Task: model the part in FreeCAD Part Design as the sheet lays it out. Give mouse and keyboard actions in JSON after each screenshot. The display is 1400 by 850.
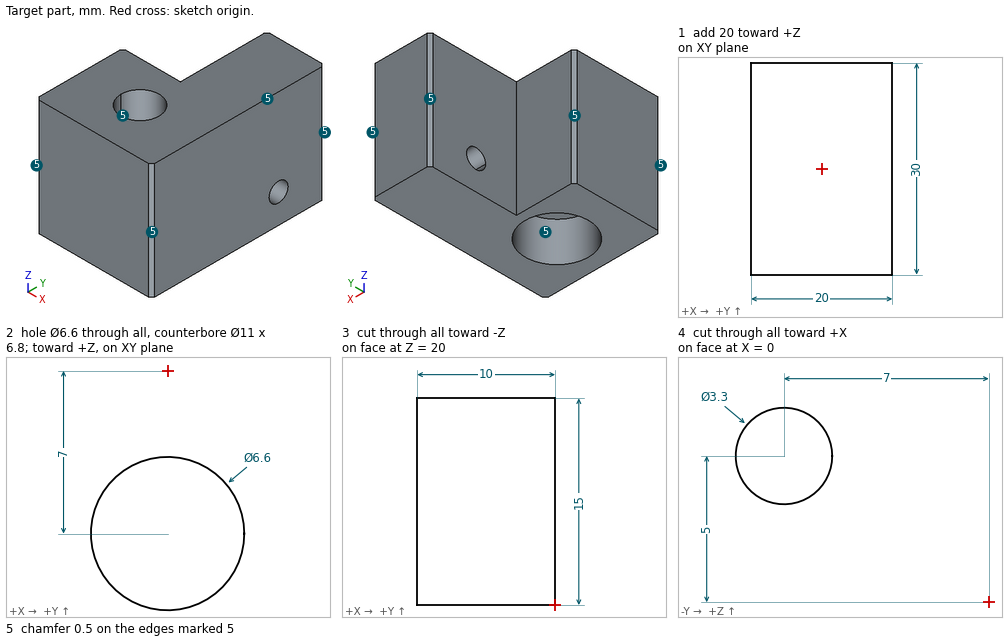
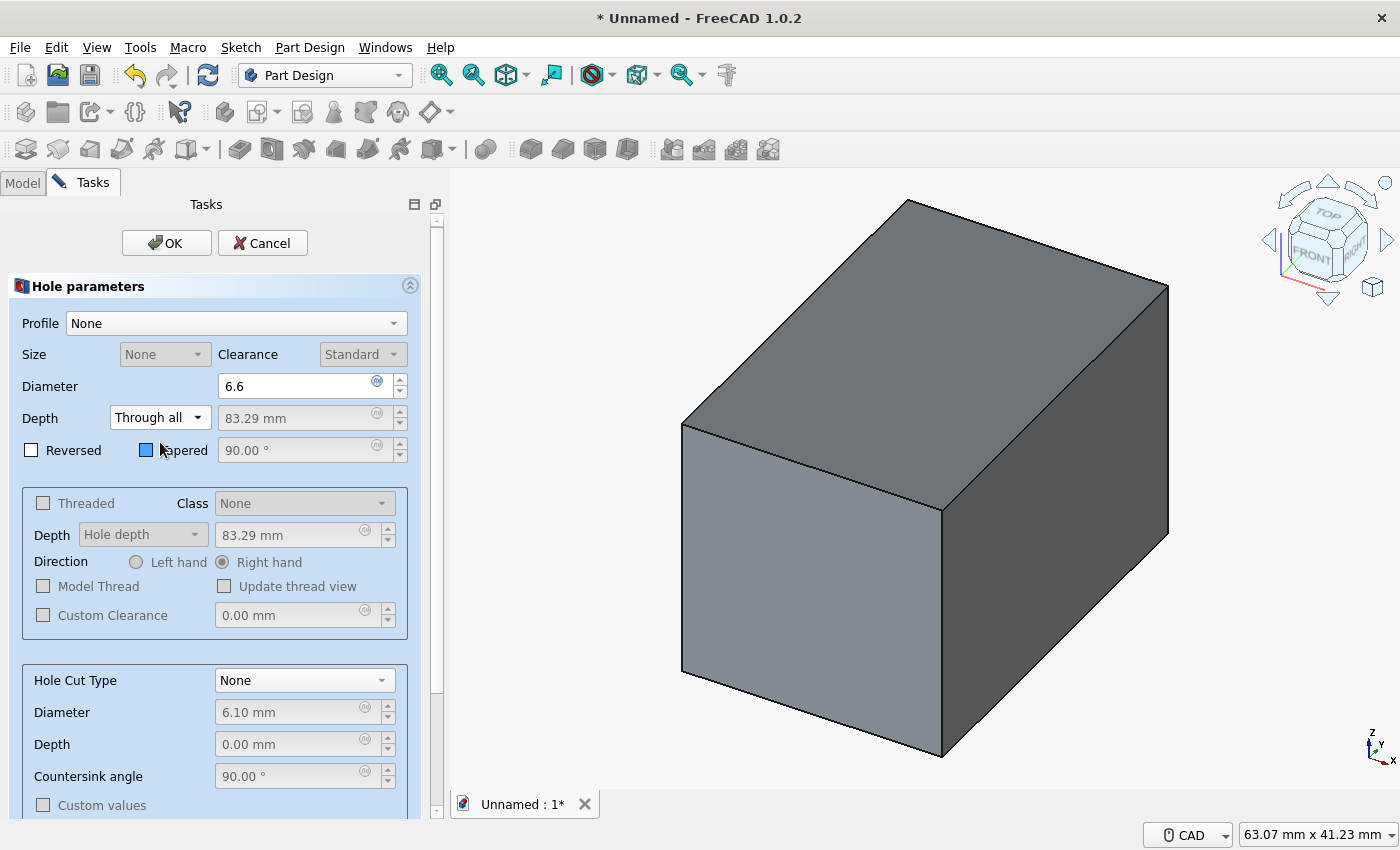
{"action": "left_click", "coordinate": [30, 450]}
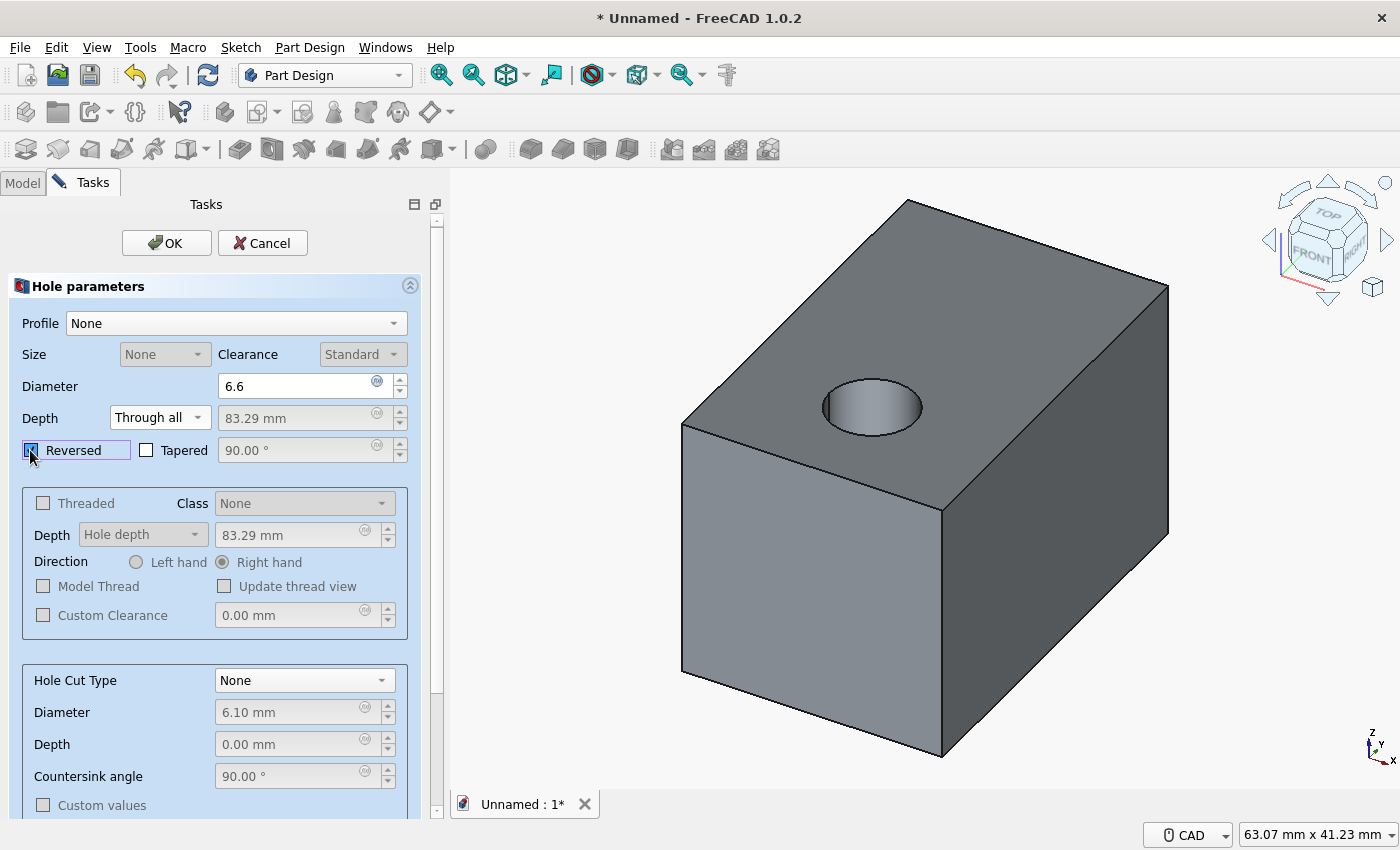
{"action": "left_click", "coordinate": [306, 680]}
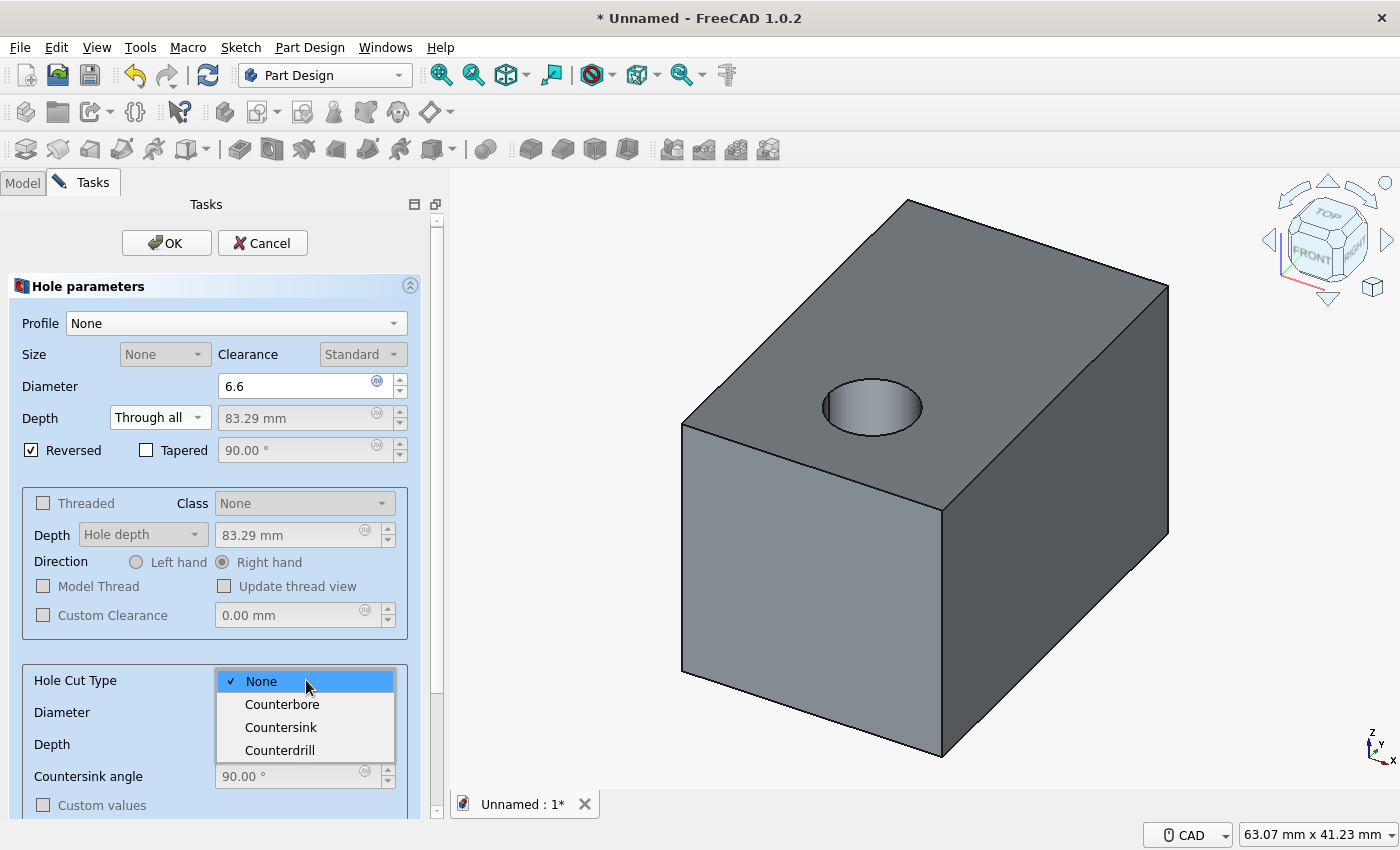
{"action": "left_click", "coordinate": [304, 704]}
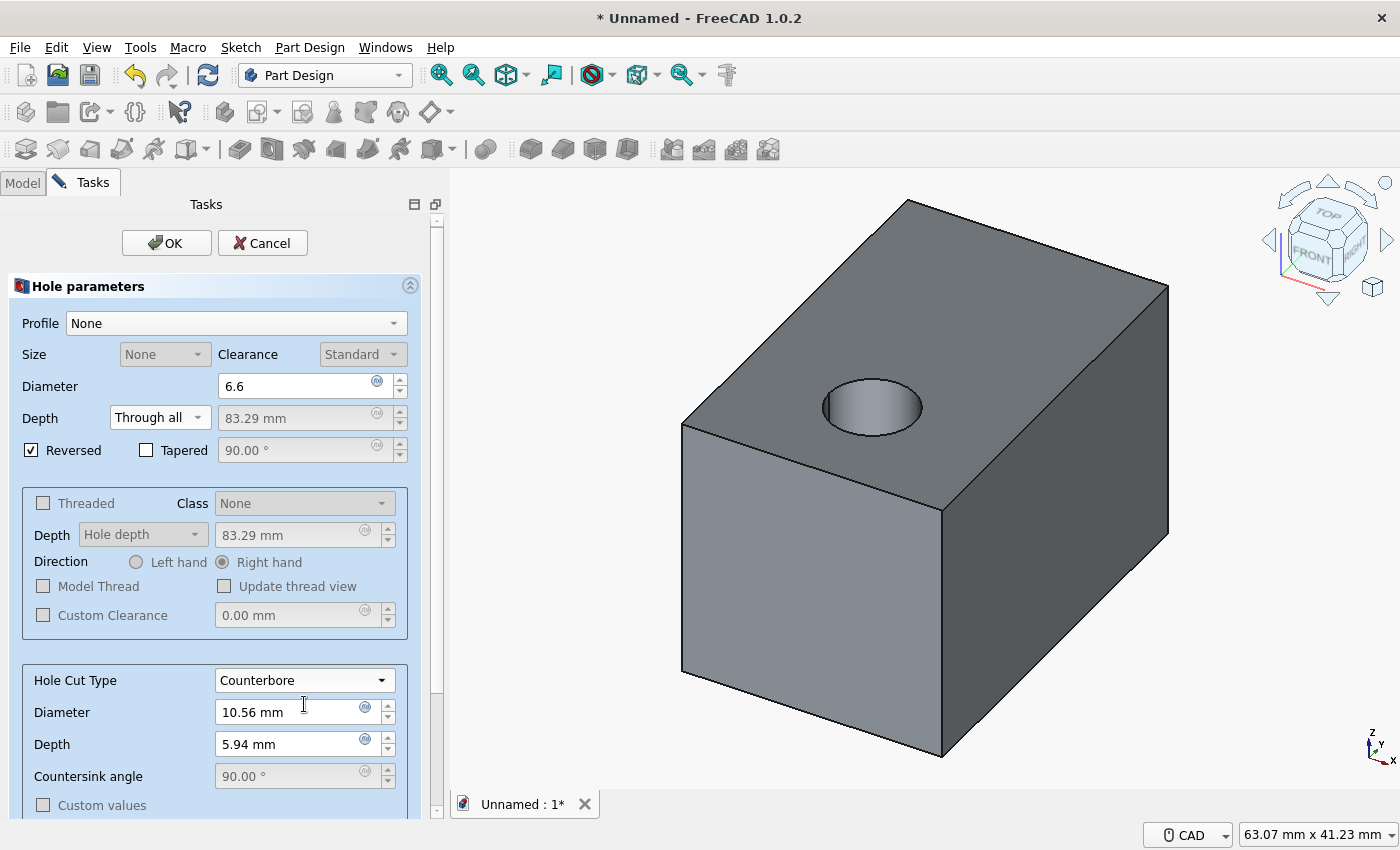
{"action": "triple_click", "coordinate": [298, 712]}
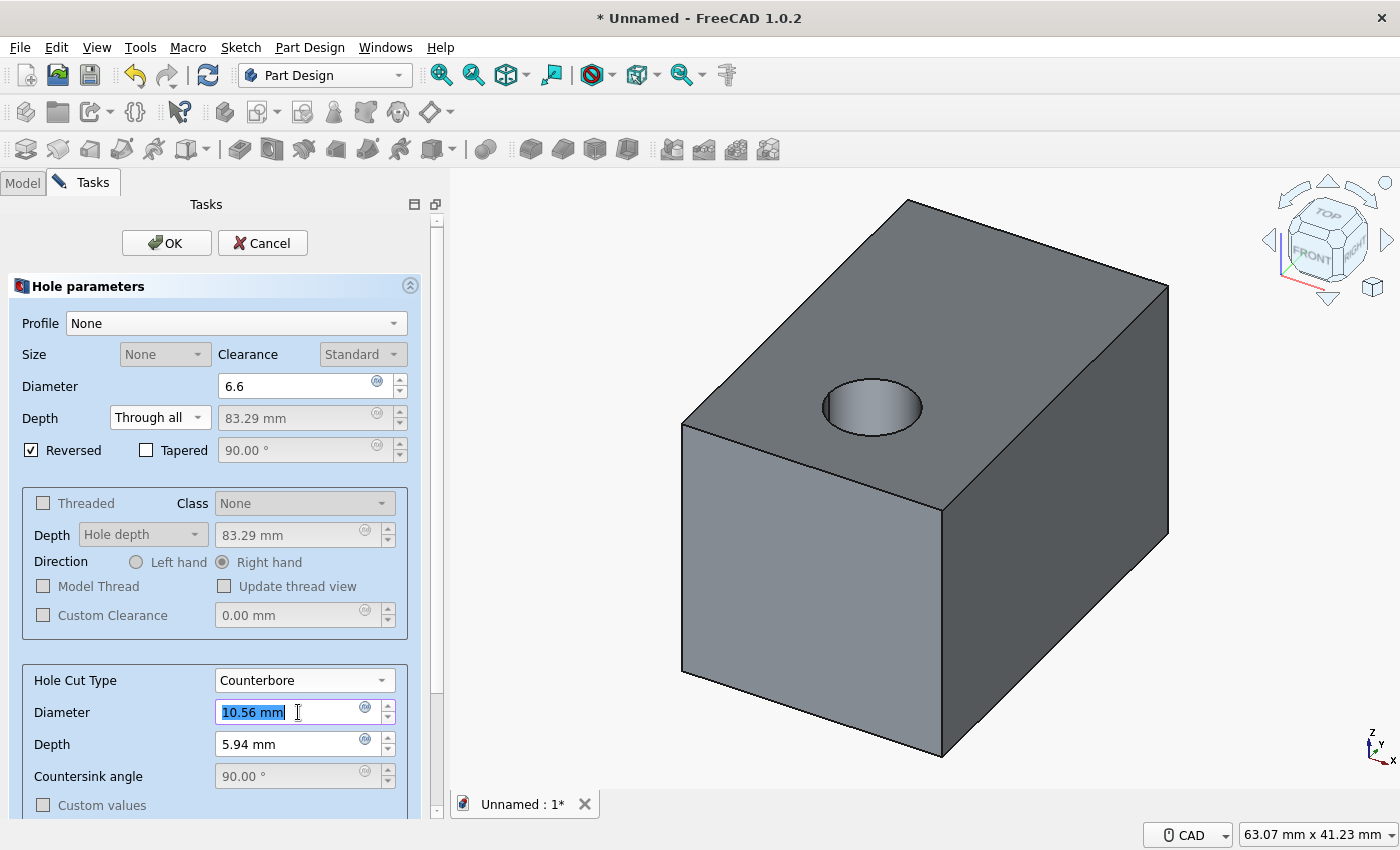
{"action": "type", "text": "11"}
{"action": "key", "text": "Tab"}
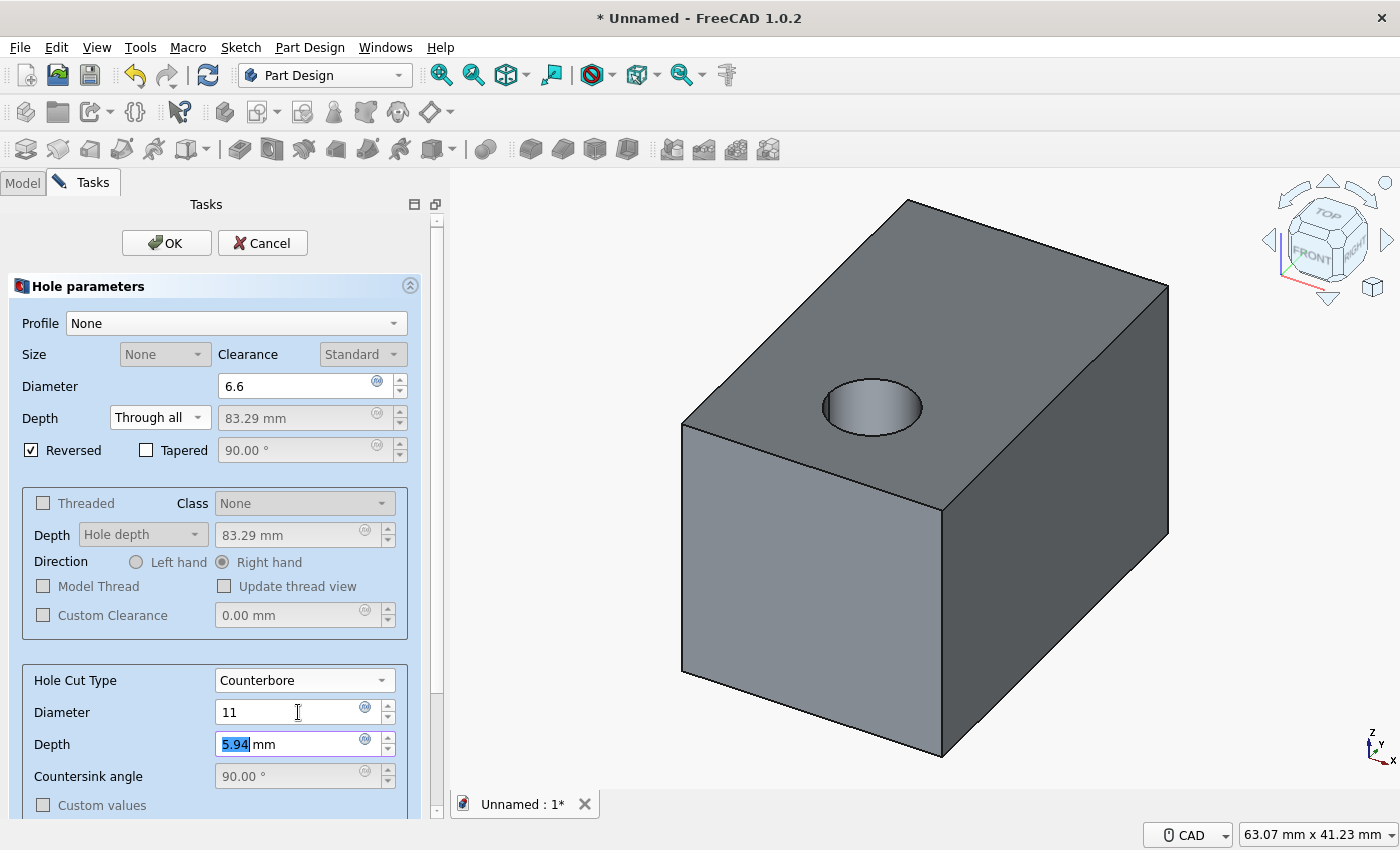
{"action": "type", "text": "6.8"}
{"action": "key", "text": "Tab"}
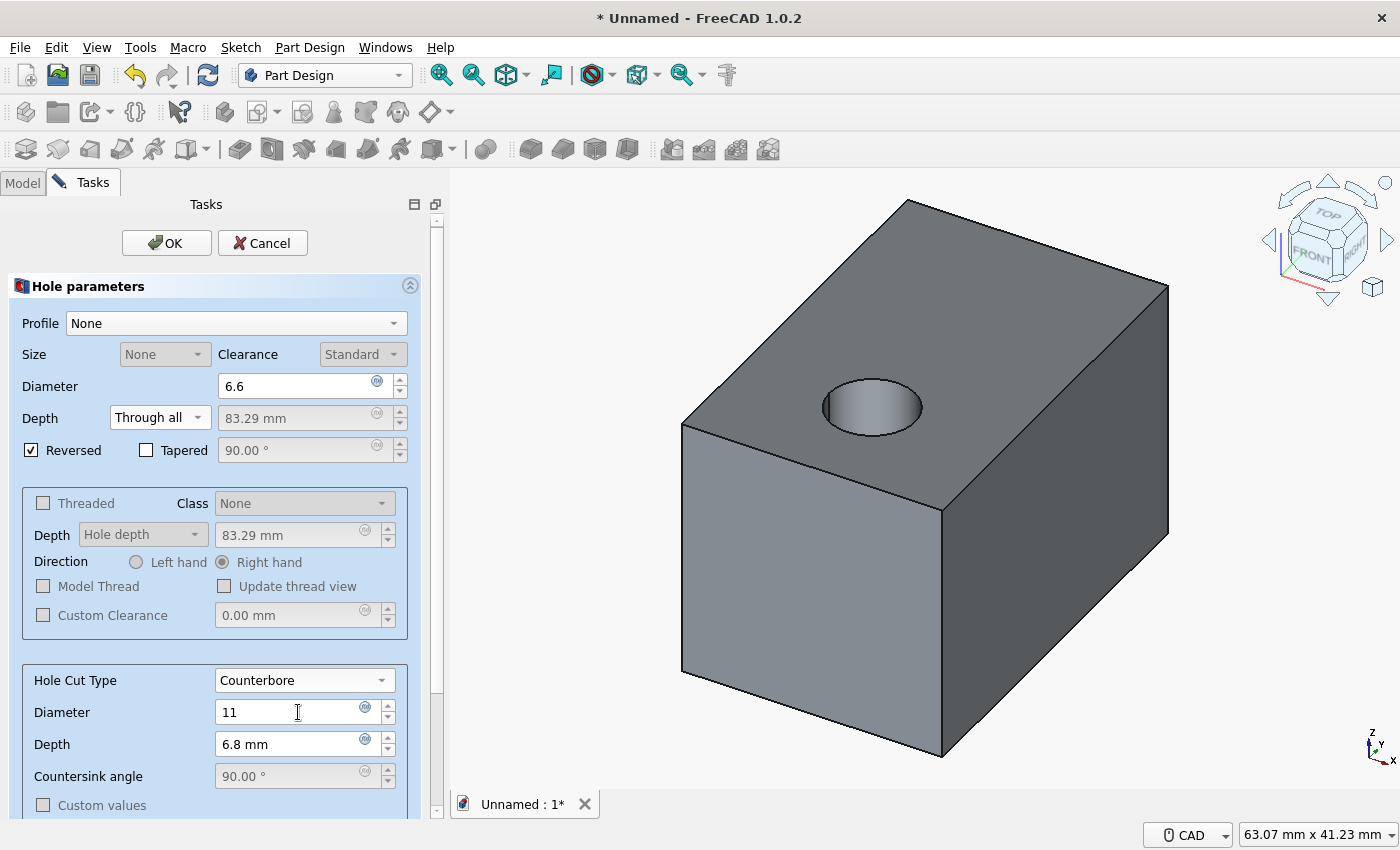
{"action": "left_click", "coordinate": [167, 243]}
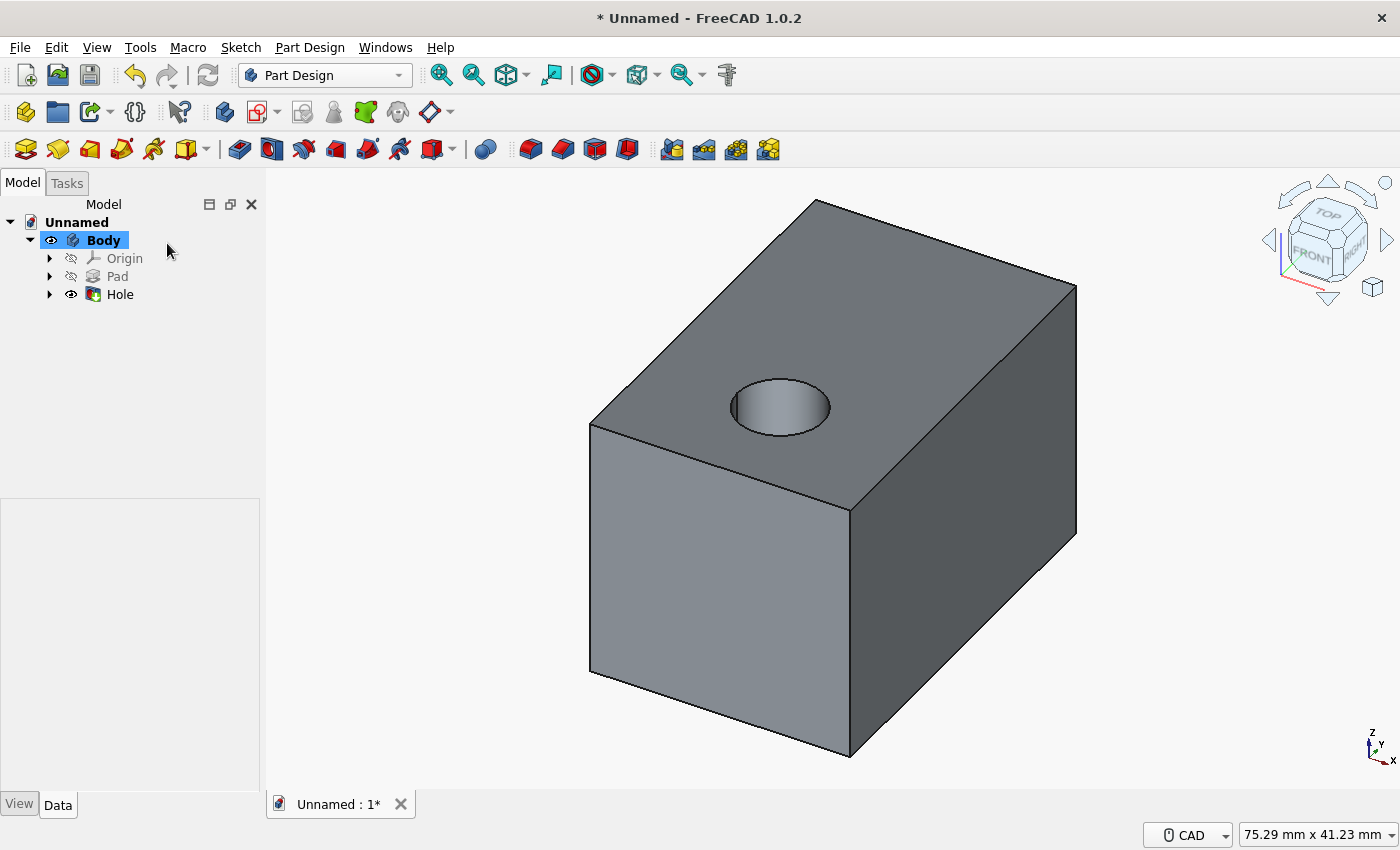
{"action": "left_click", "coordinate": [865, 322]}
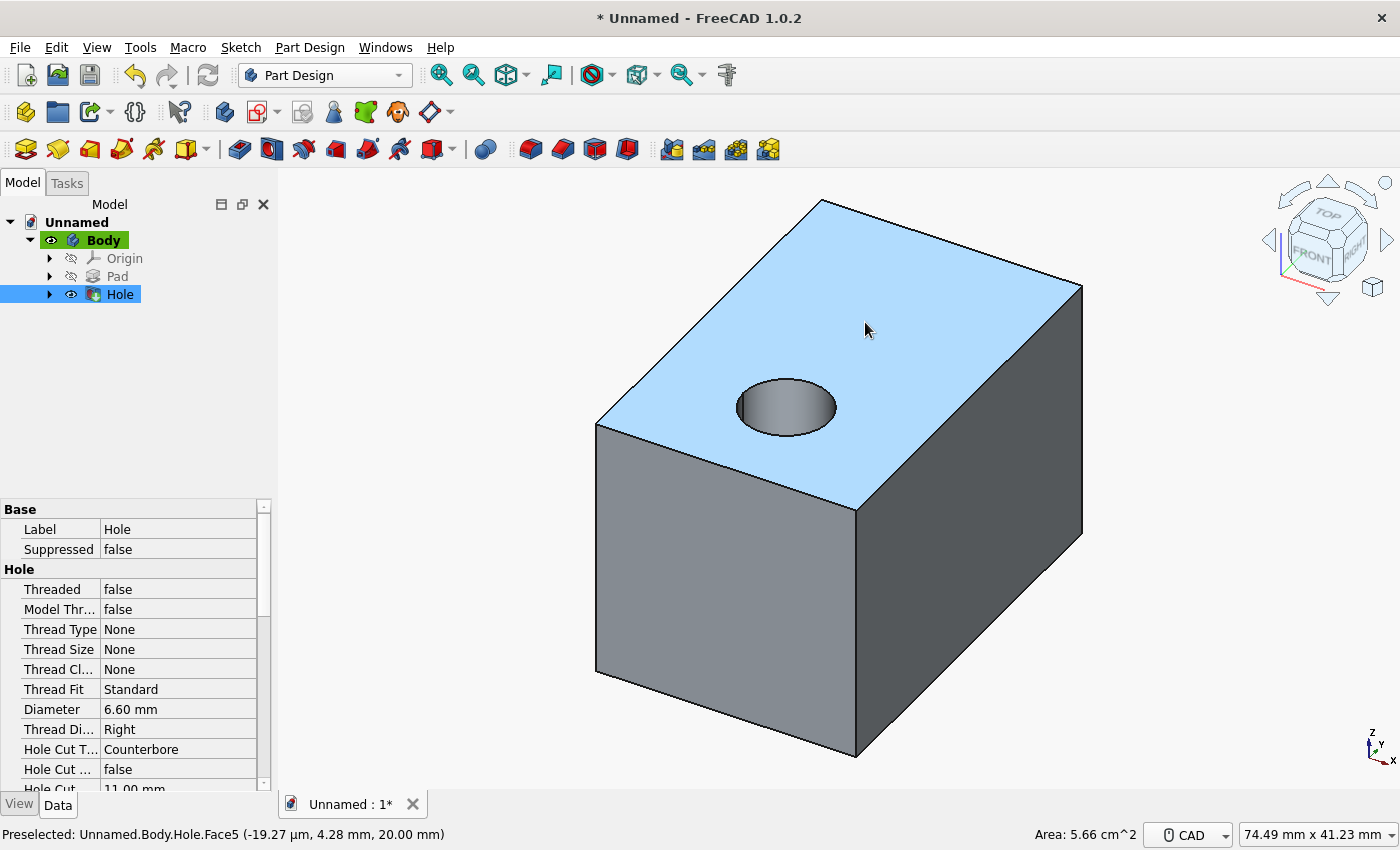
{"action": "left_click", "coordinate": [258, 112]}